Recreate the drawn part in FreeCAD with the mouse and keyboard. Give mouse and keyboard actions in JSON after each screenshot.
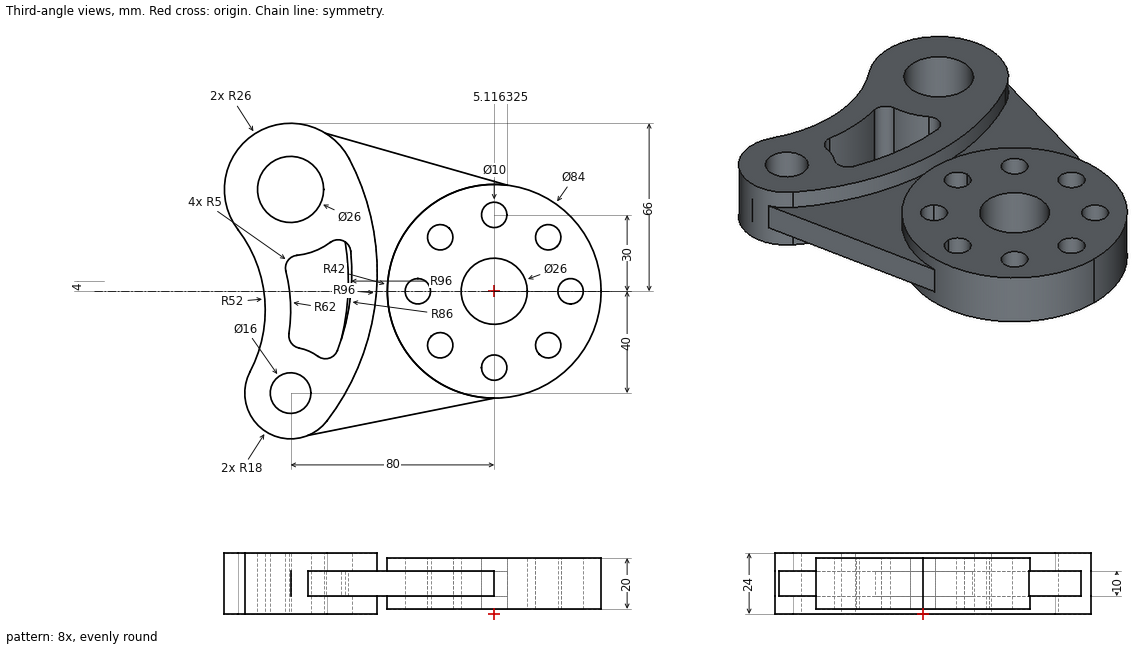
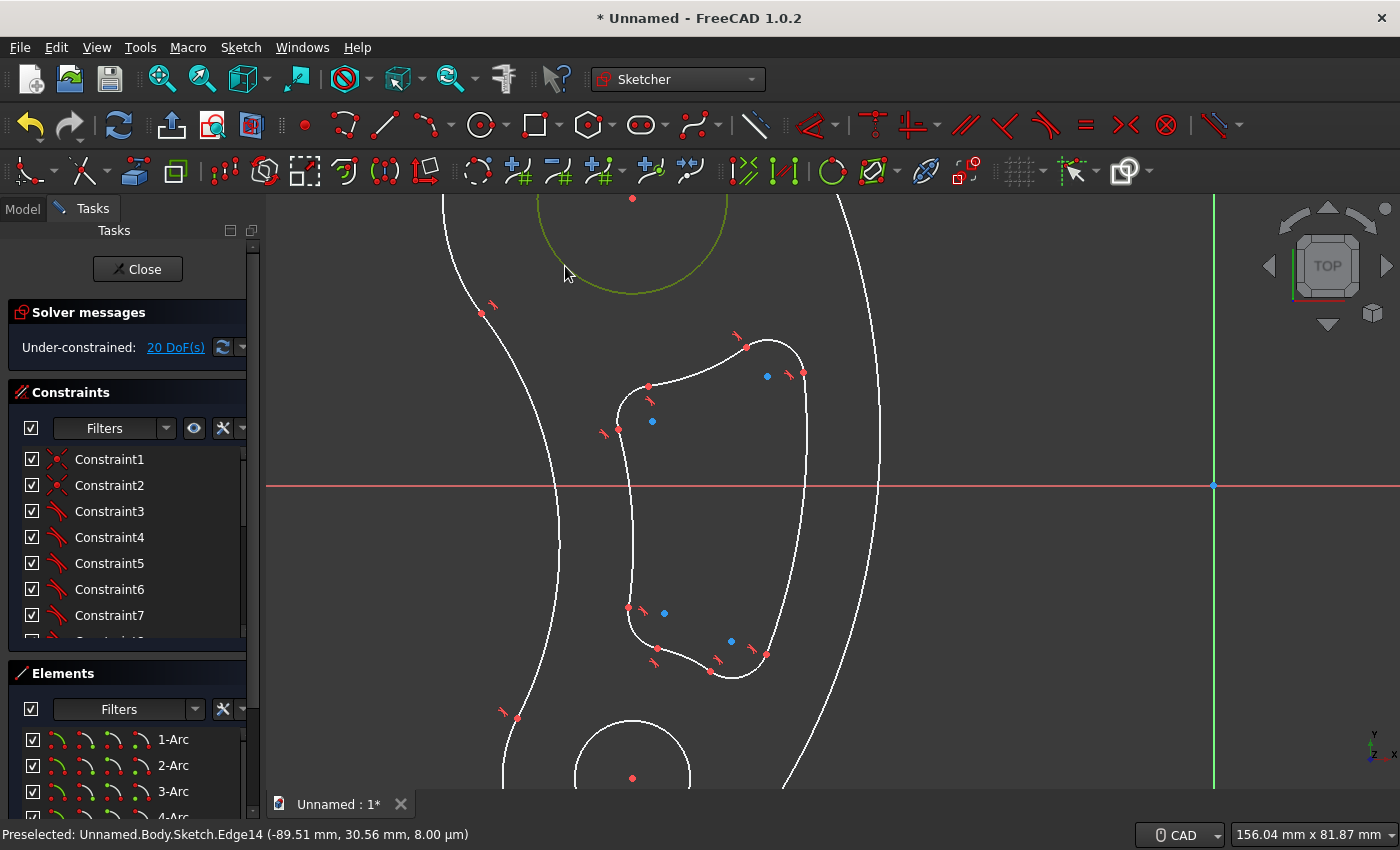
{"action": "left_click", "coordinate": [679, 380]}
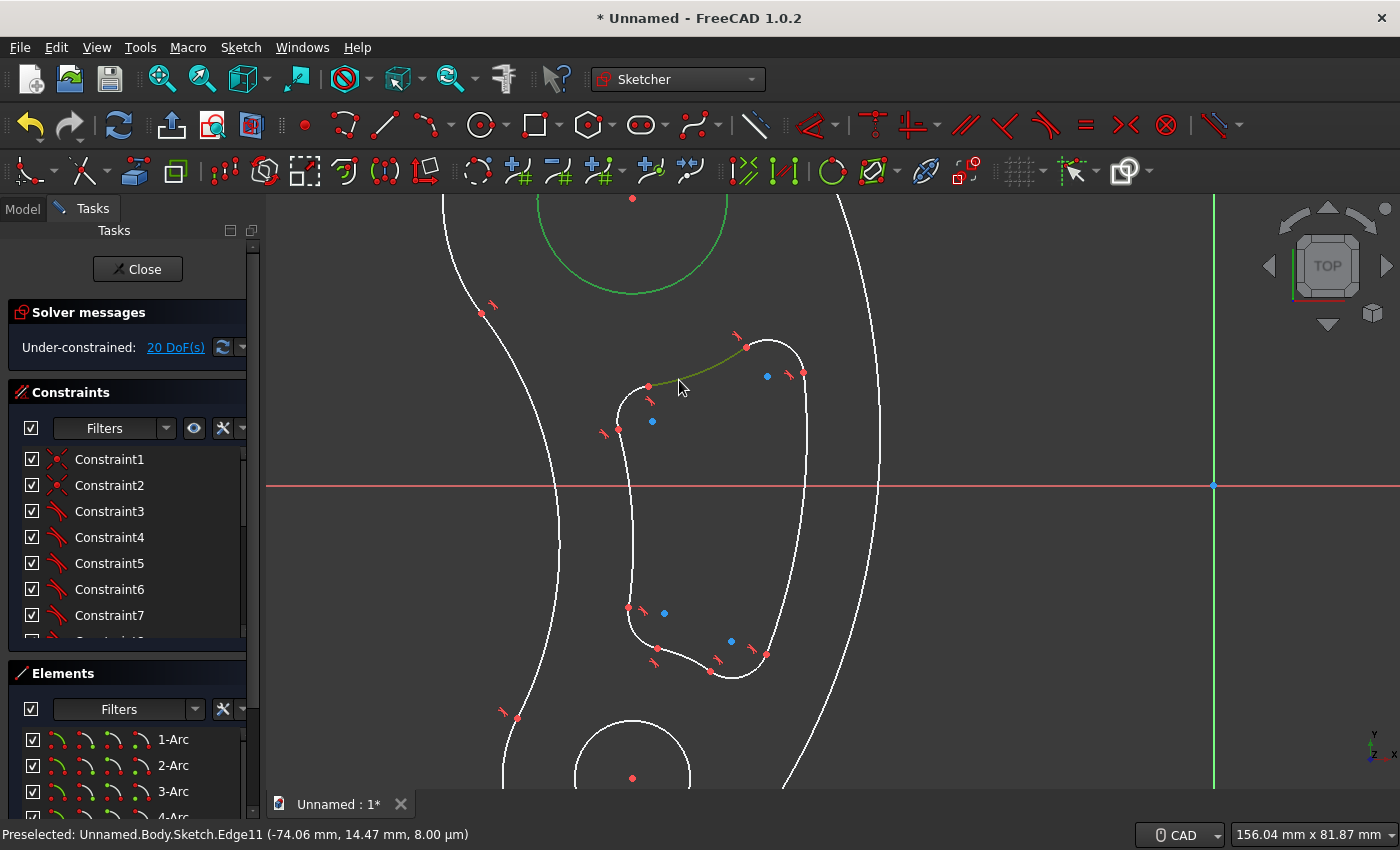
{"action": "left_click", "coordinate": [874, 126]}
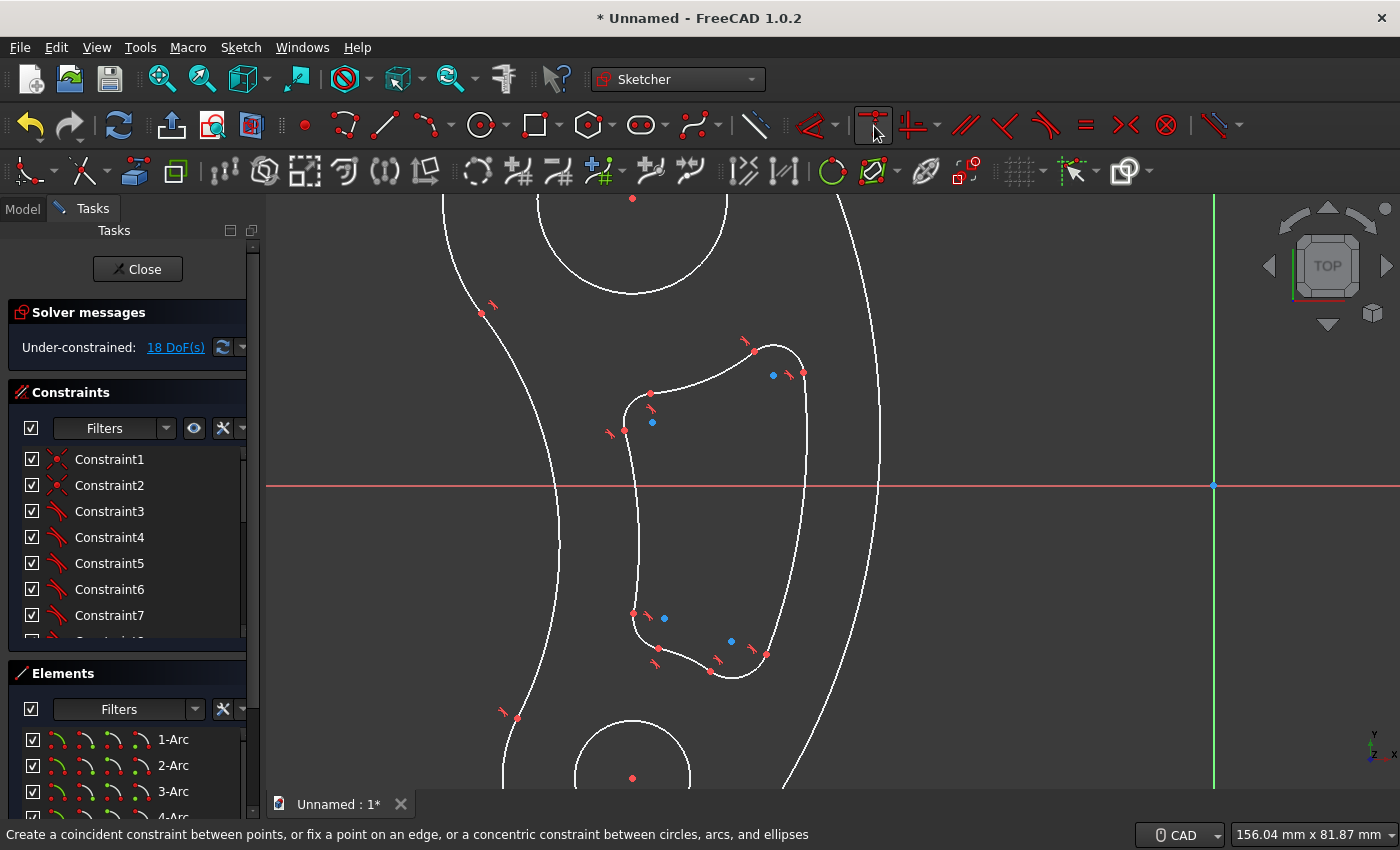
{"action": "scroll", "coordinate": [696, 516], "scroll_direction": "down", "scroll_amount": 4}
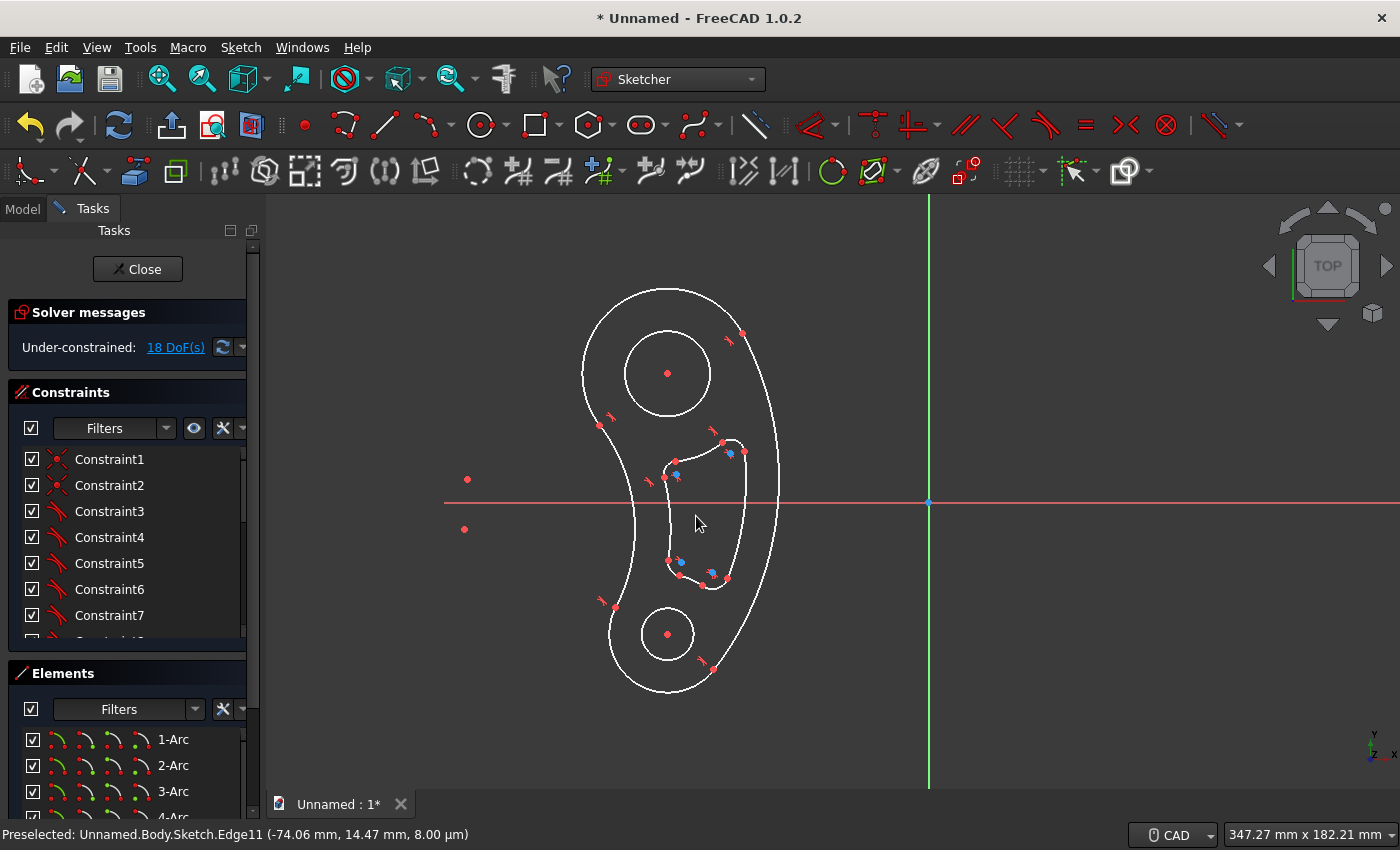
{"action": "left_click", "coordinate": [614, 658]}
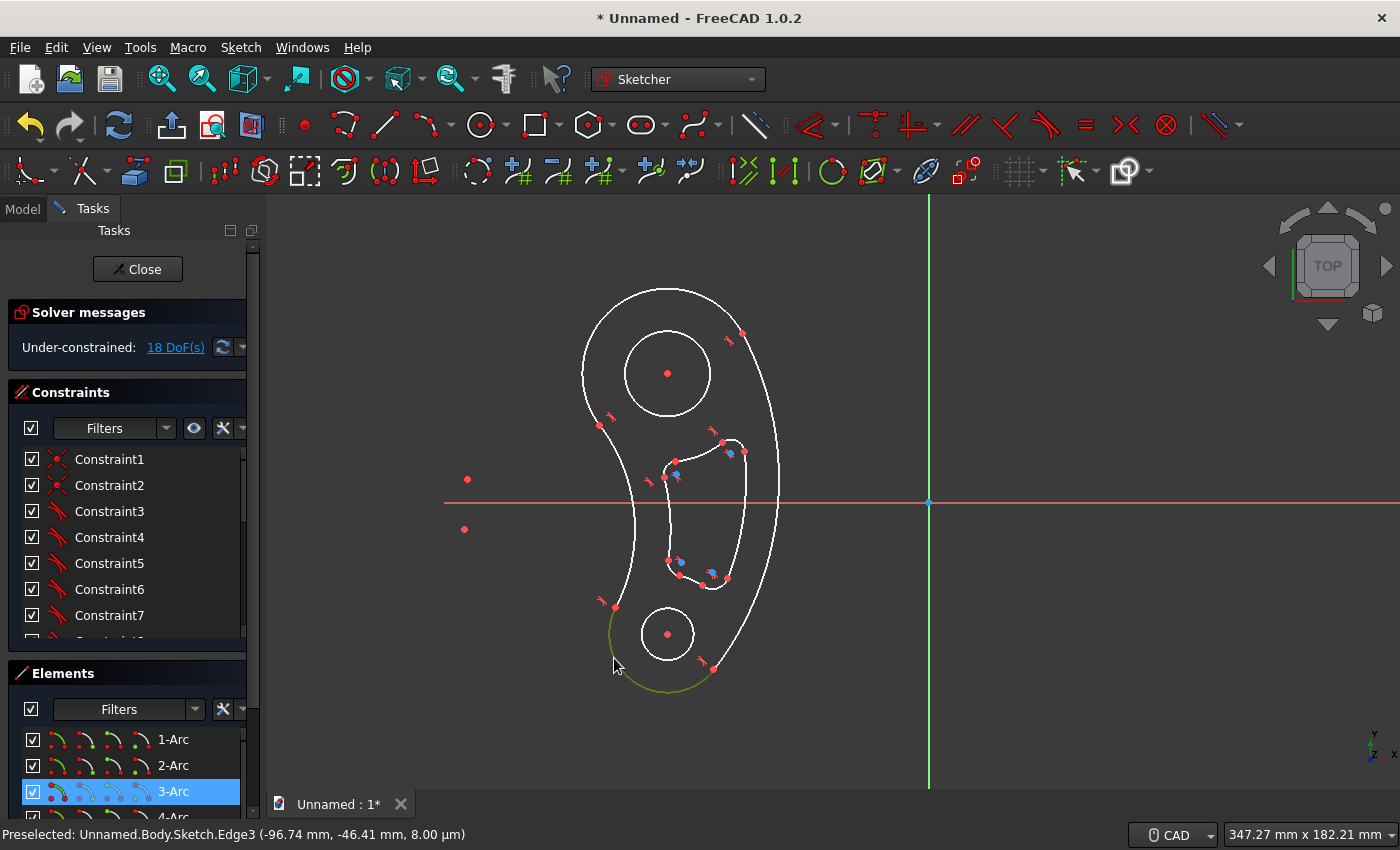
{"action": "left_click", "coordinate": [691, 580]}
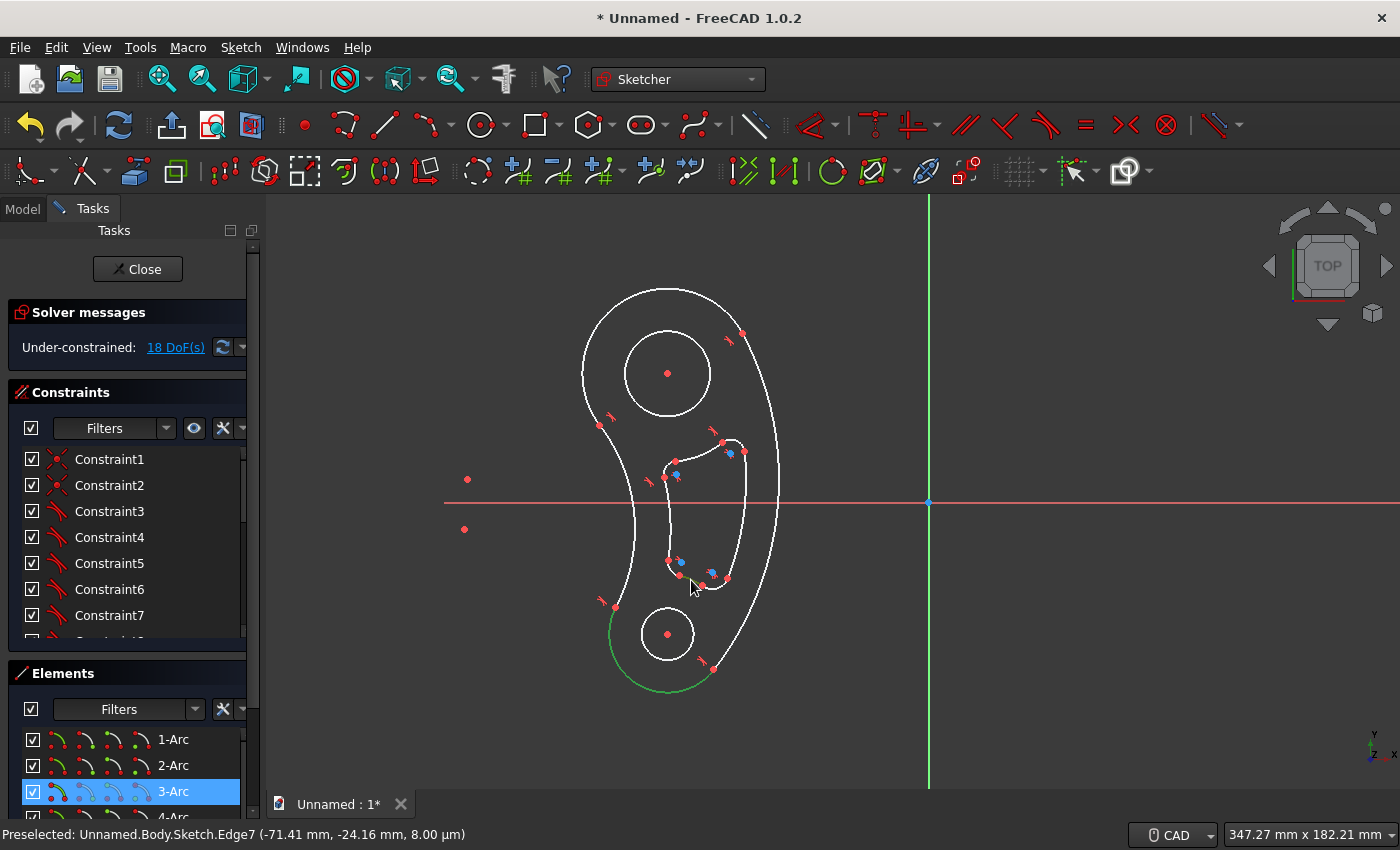
{"action": "left_click", "coordinate": [1086, 126]}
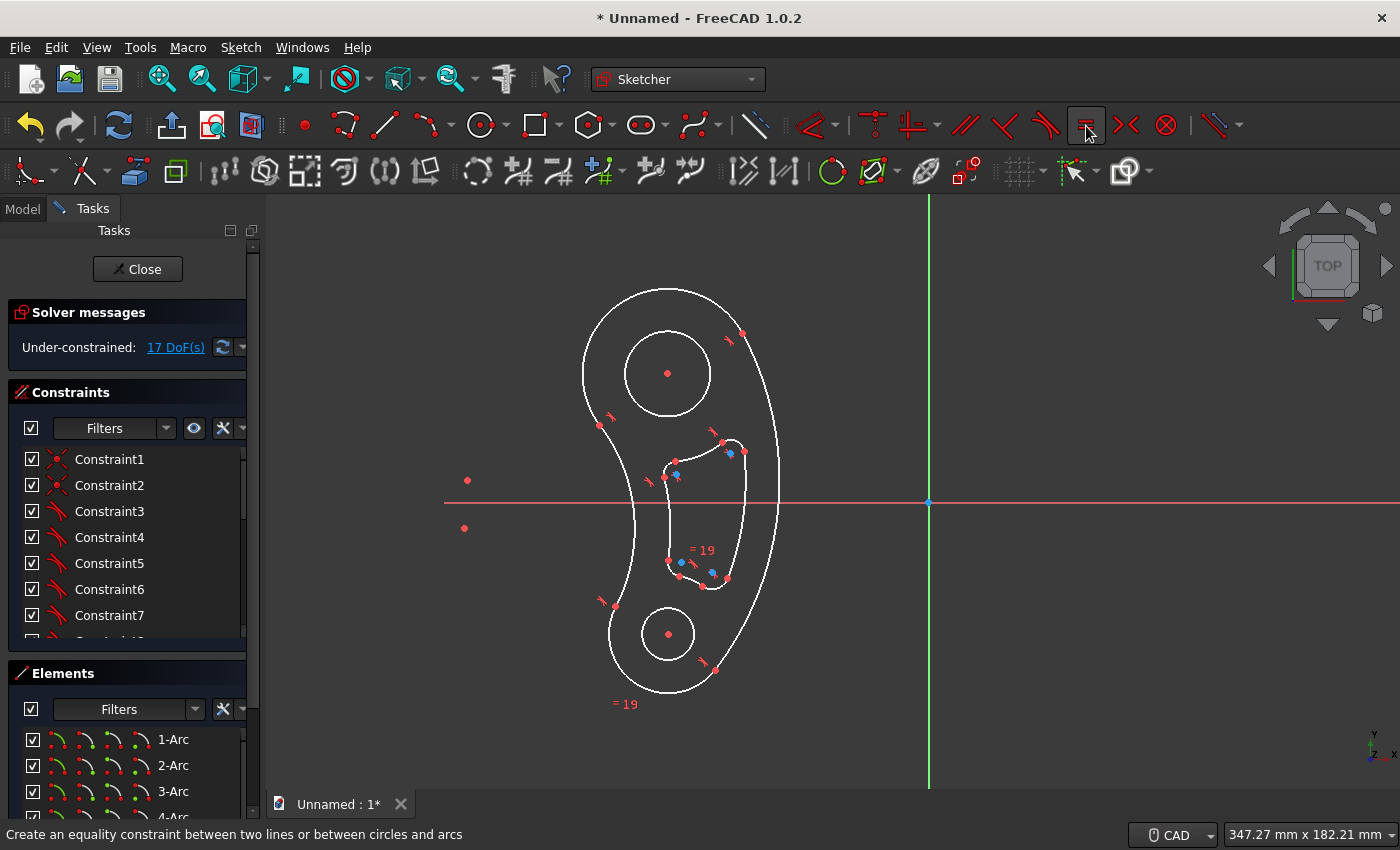
{"action": "scroll", "coordinate": [711, 589], "scroll_direction": "up", "scroll_amount": 3}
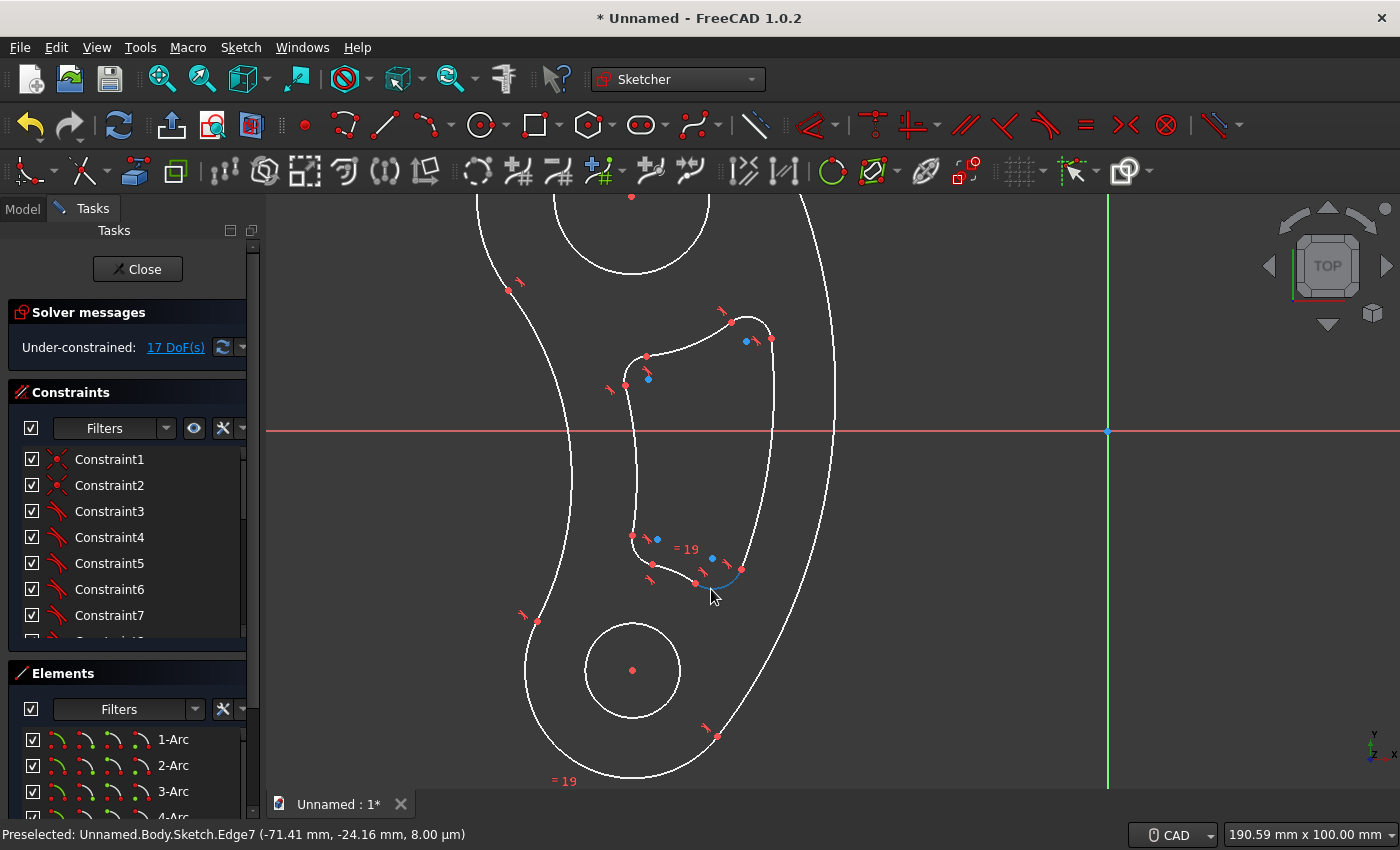
{"action": "left_click", "coordinate": [711, 589]}